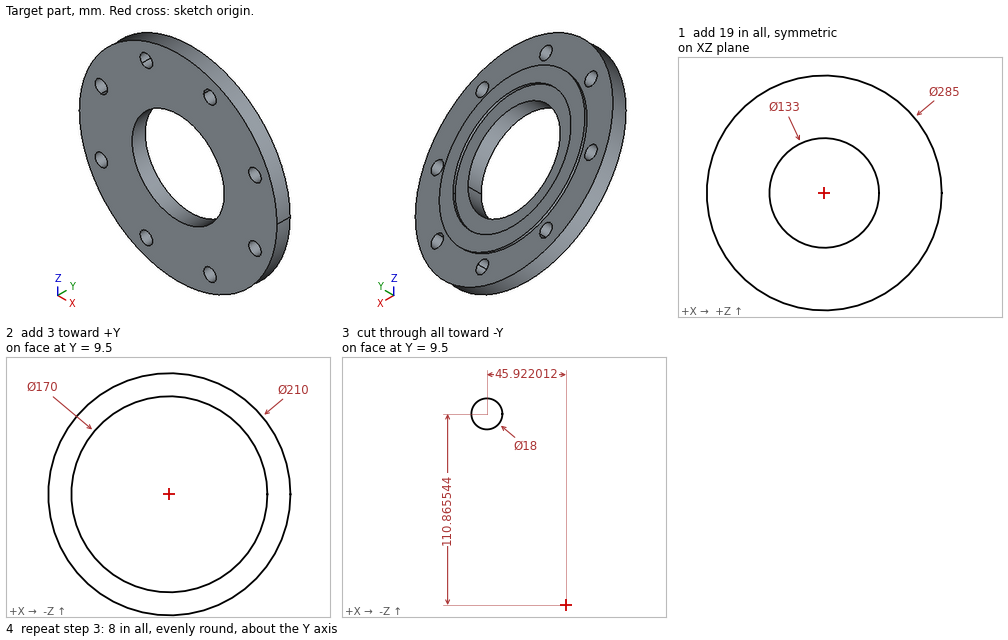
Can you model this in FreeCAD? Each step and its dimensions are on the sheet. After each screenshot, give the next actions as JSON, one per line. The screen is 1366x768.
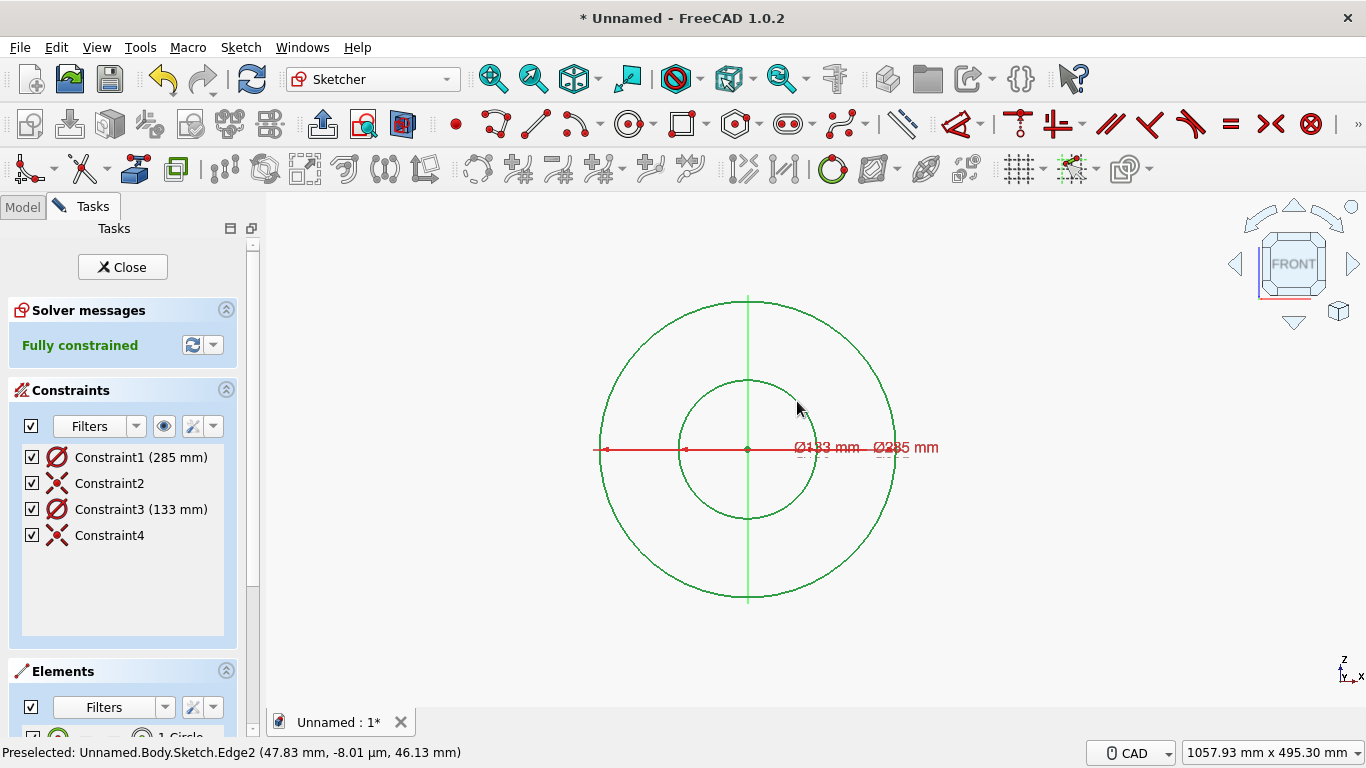
{"action": "left_click", "coordinate": [123, 267]}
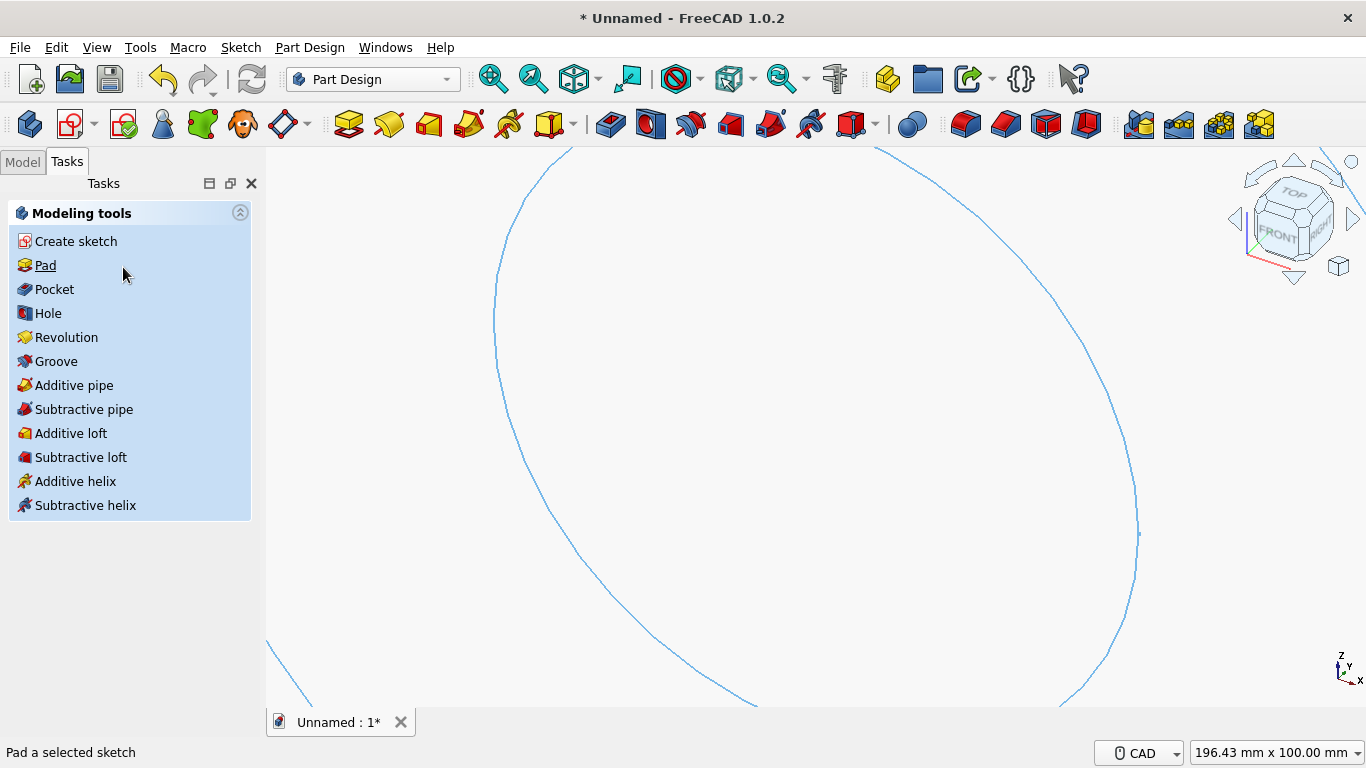
{"action": "left_click", "coordinate": [350, 124]}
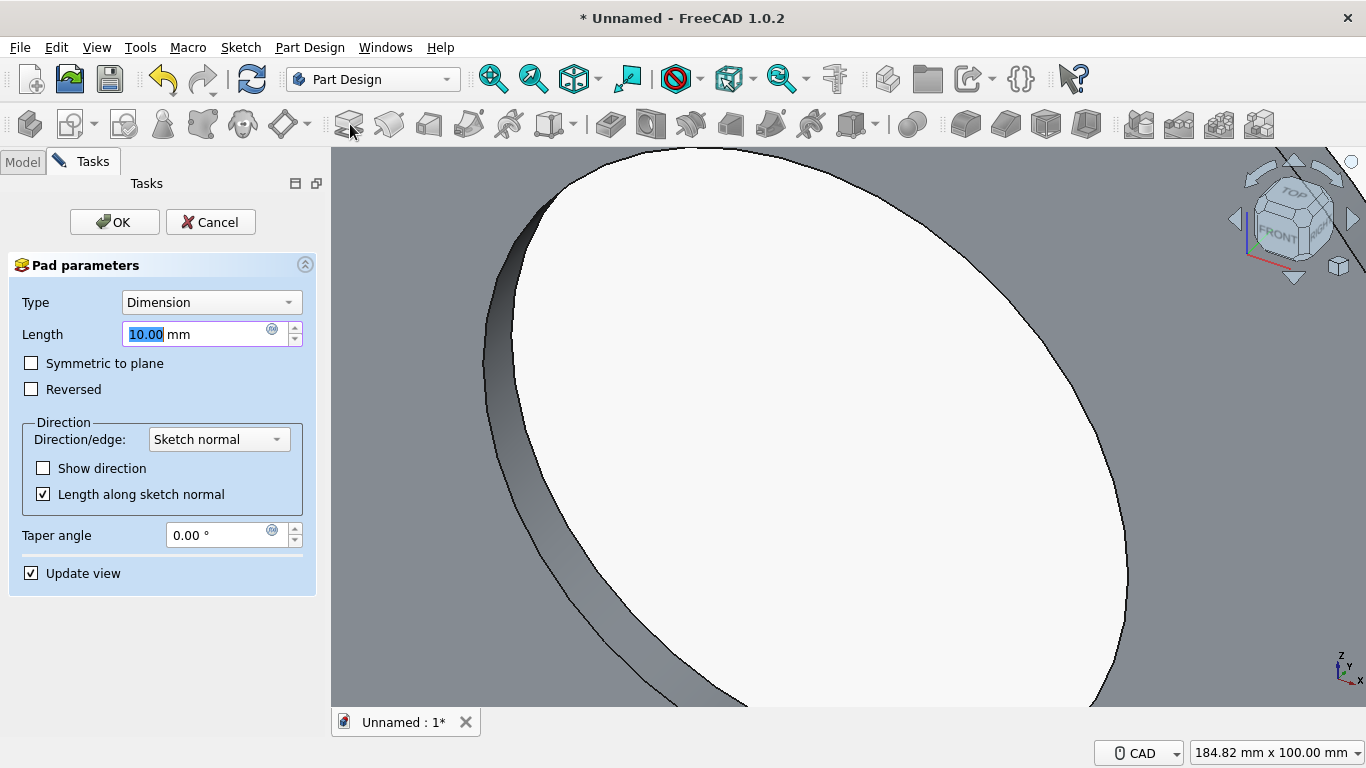
{"action": "type", "text": "19"}
{"action": "key", "text": "Tab"}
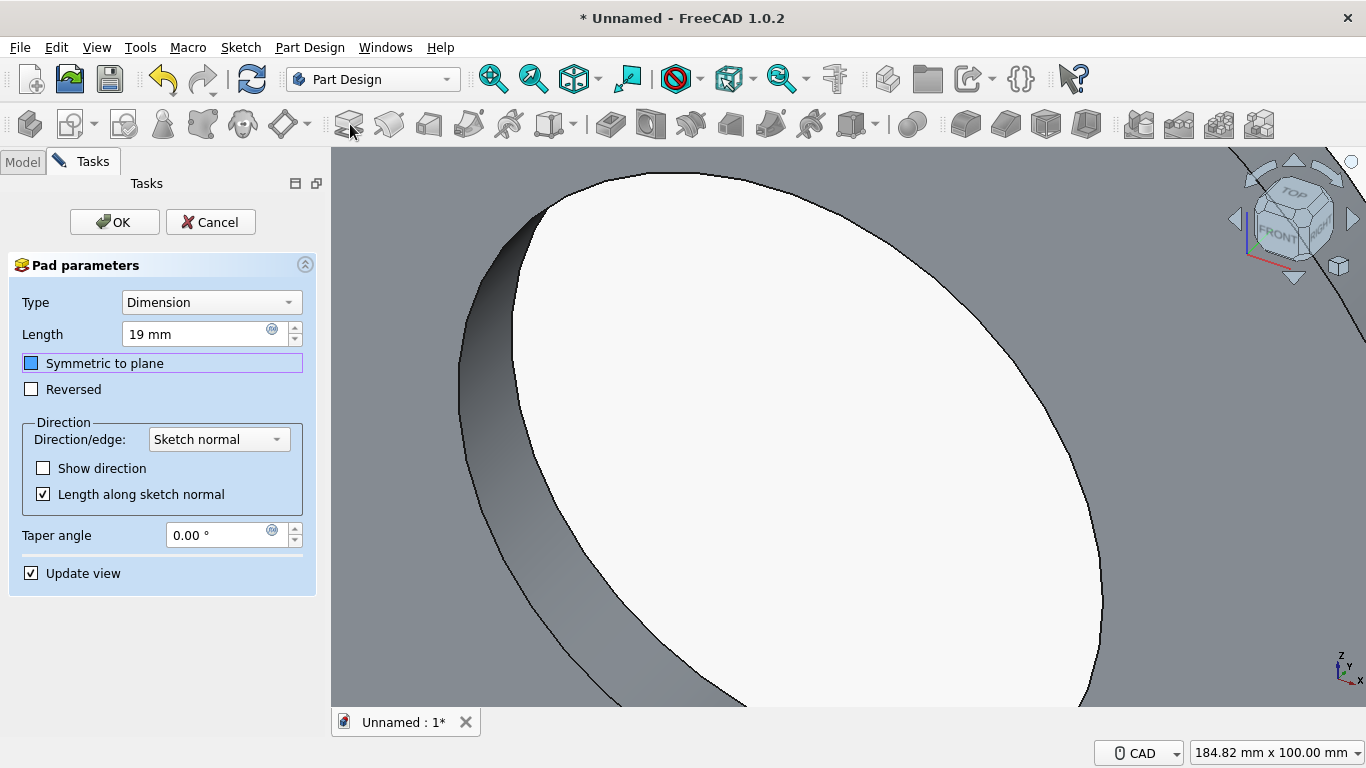
{"action": "left_click", "coordinate": [30, 363]}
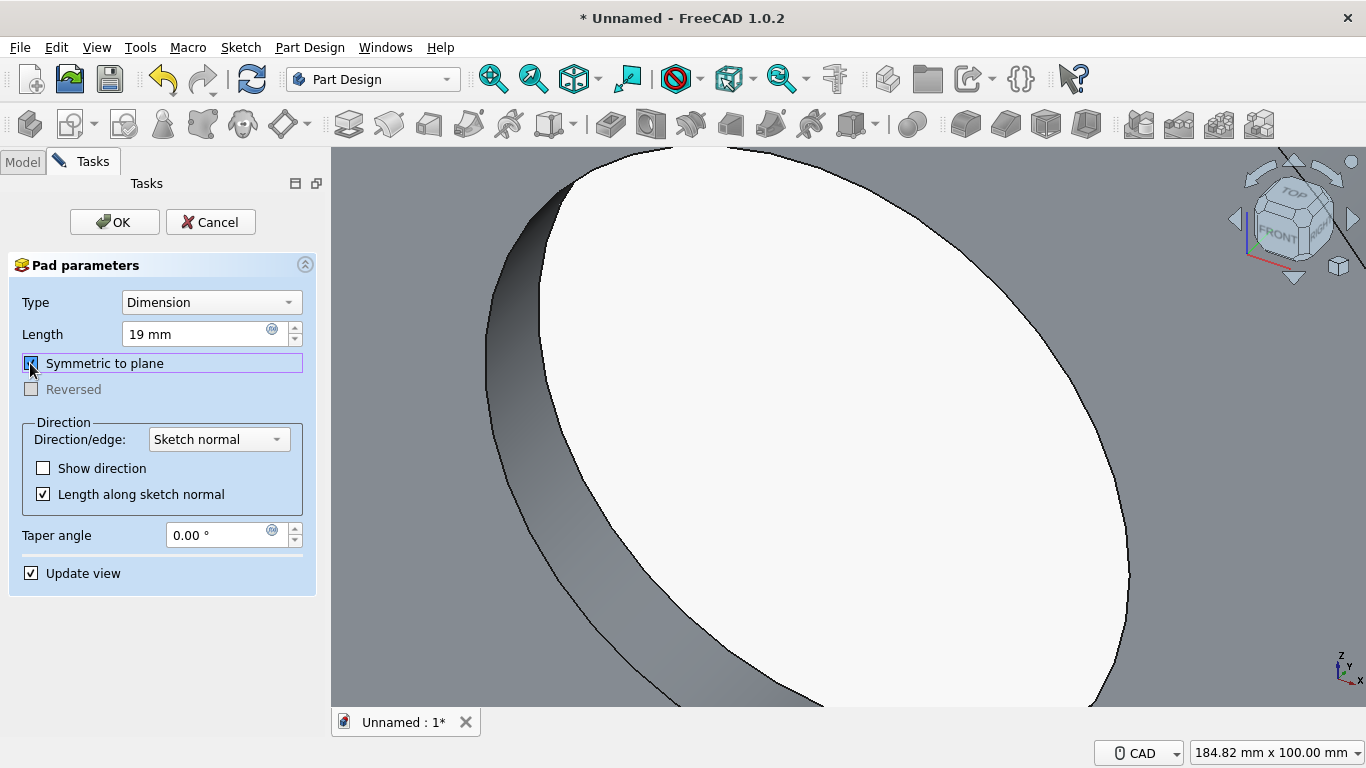
{"action": "left_click", "coordinate": [115, 222]}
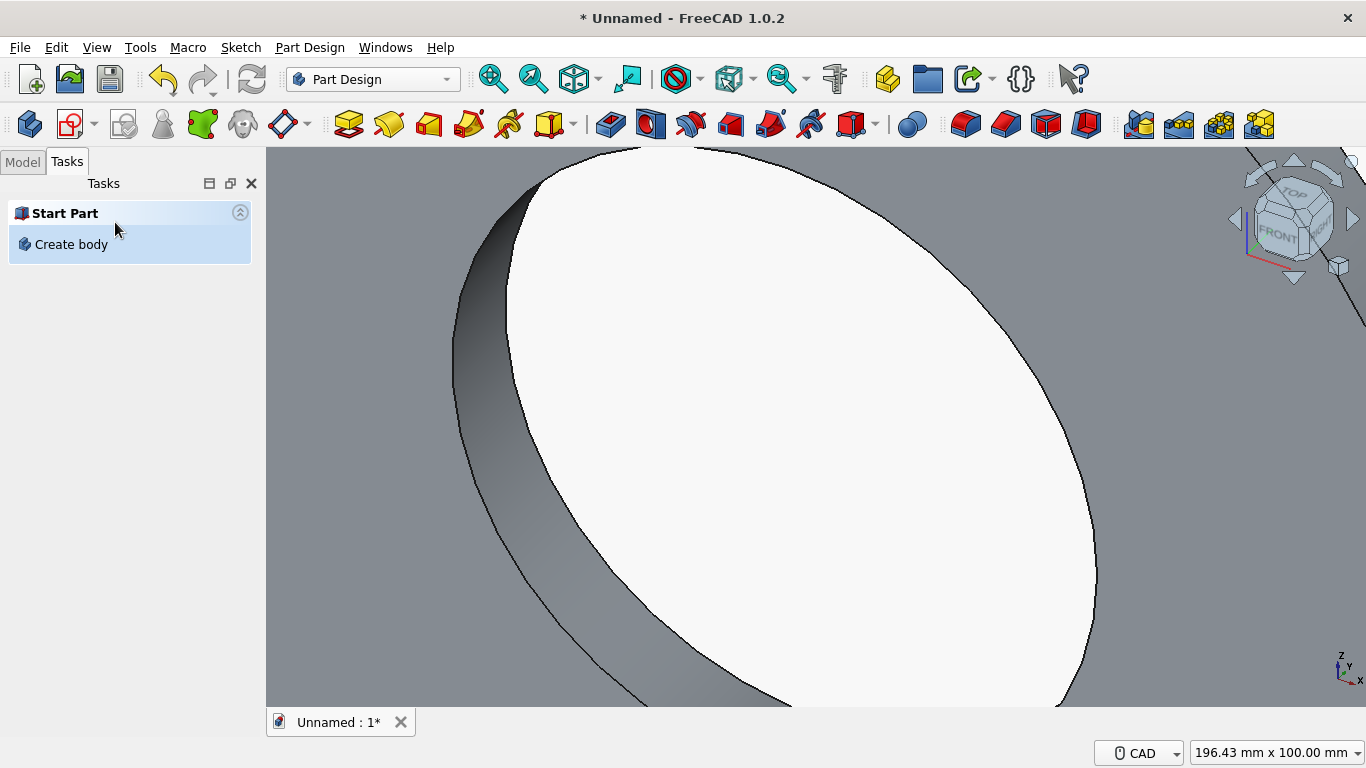
{"action": "left_click", "coordinate": [494, 80]}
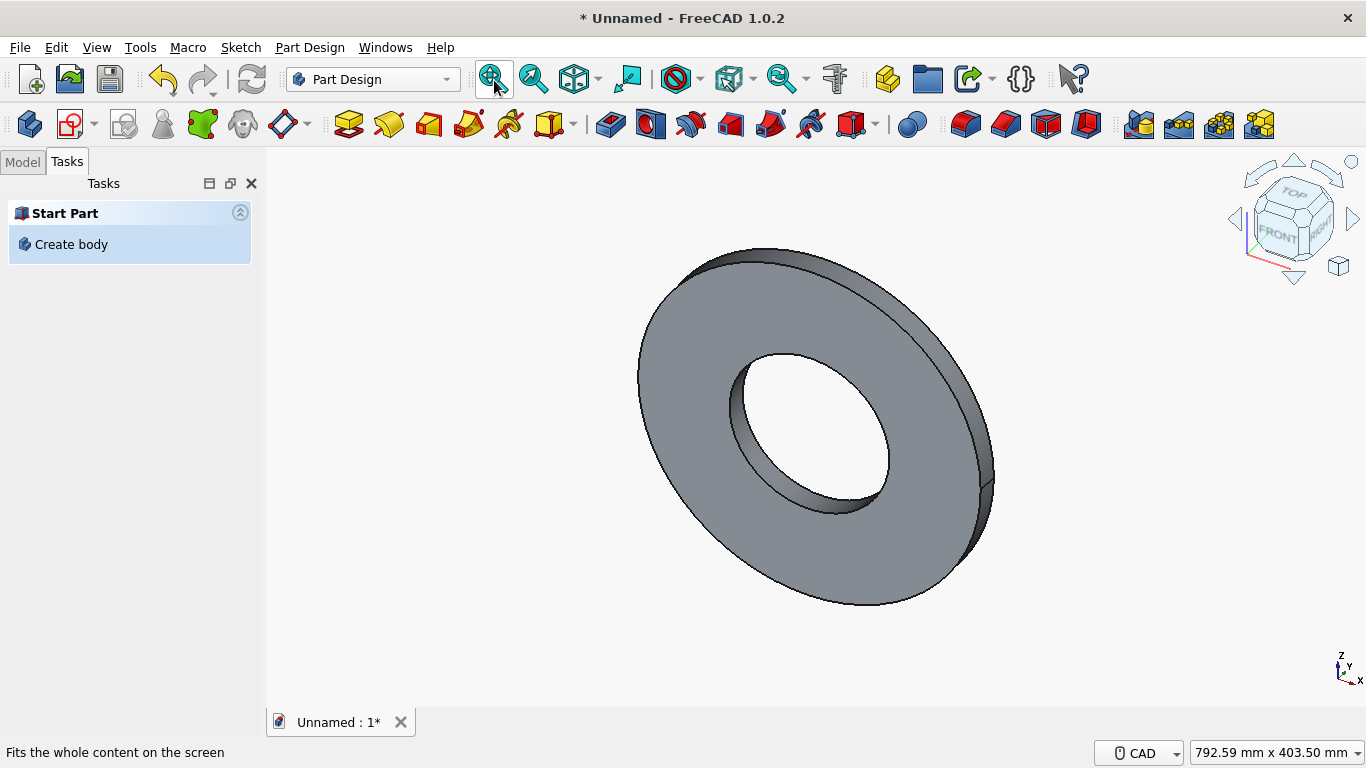
{"action": "key", "text": "4"}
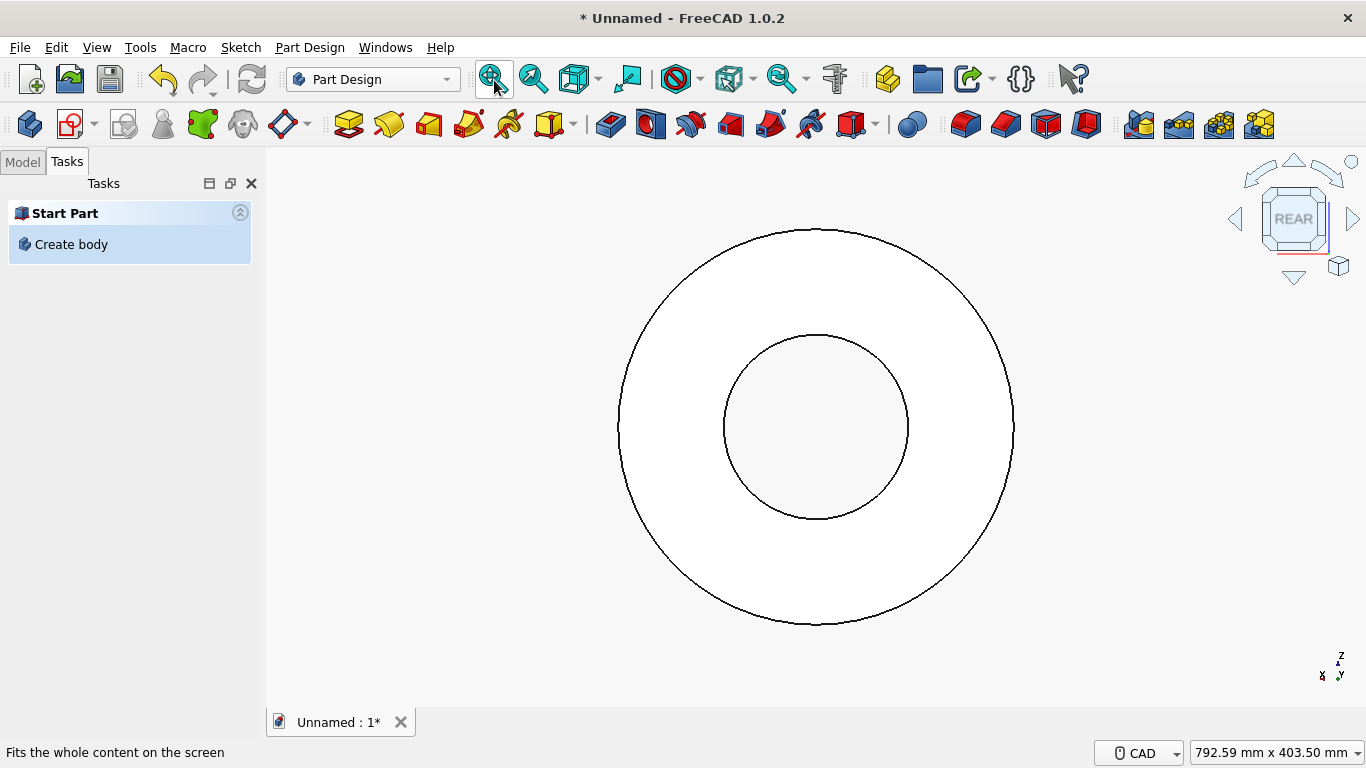
{"action": "left_click", "coordinate": [703, 313]}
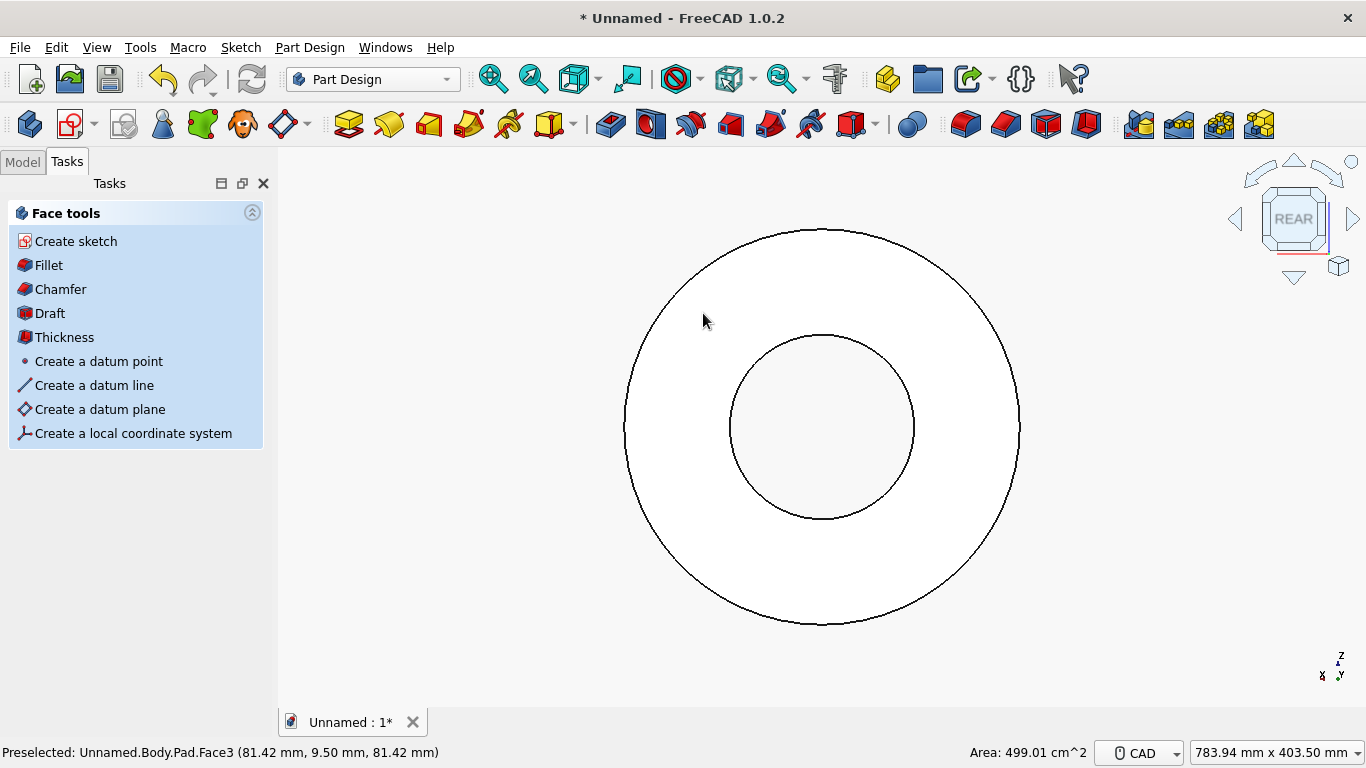
{"action": "left_click", "coordinate": [70, 124]}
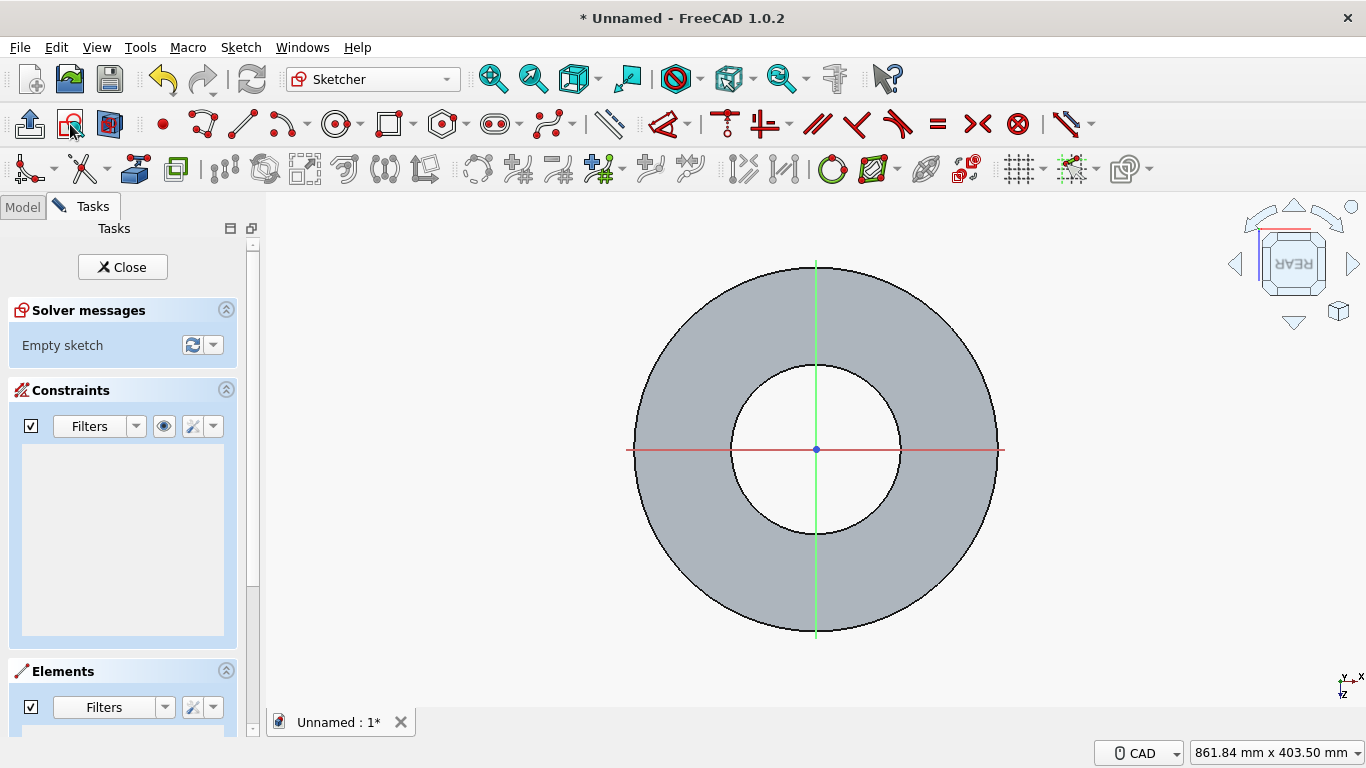
{"action": "key", "text": "g c"}